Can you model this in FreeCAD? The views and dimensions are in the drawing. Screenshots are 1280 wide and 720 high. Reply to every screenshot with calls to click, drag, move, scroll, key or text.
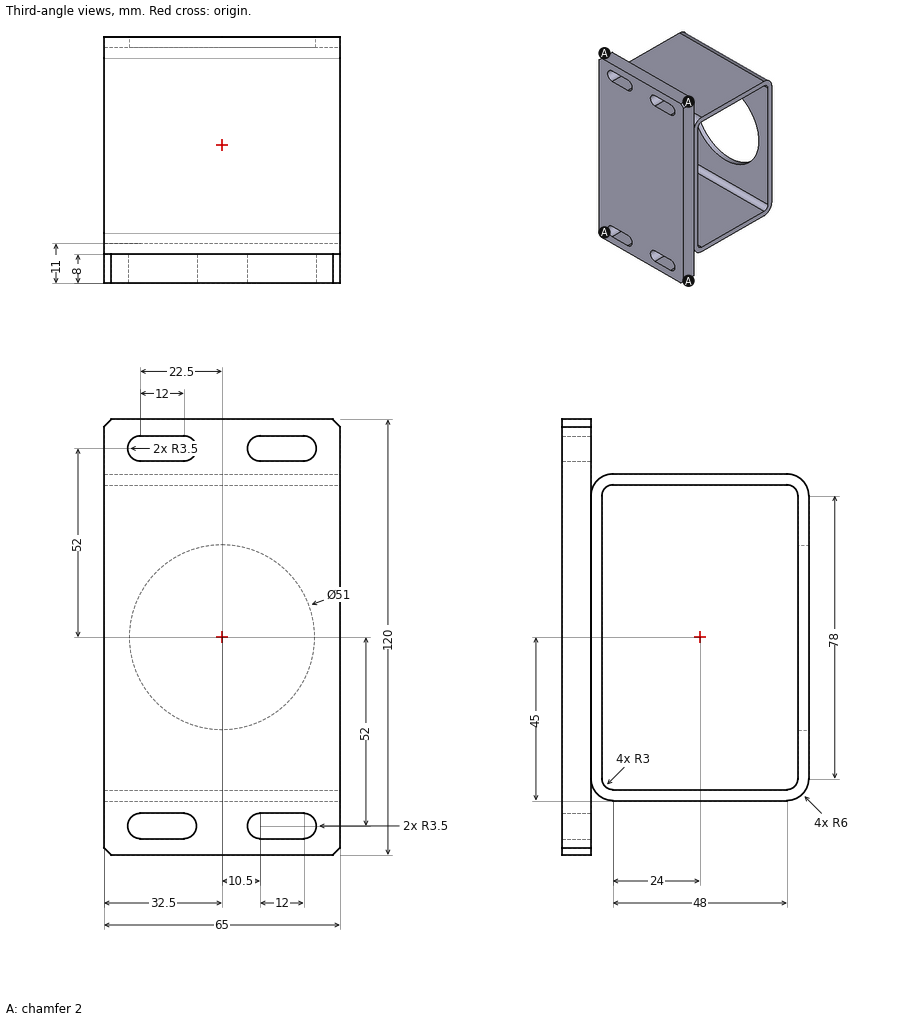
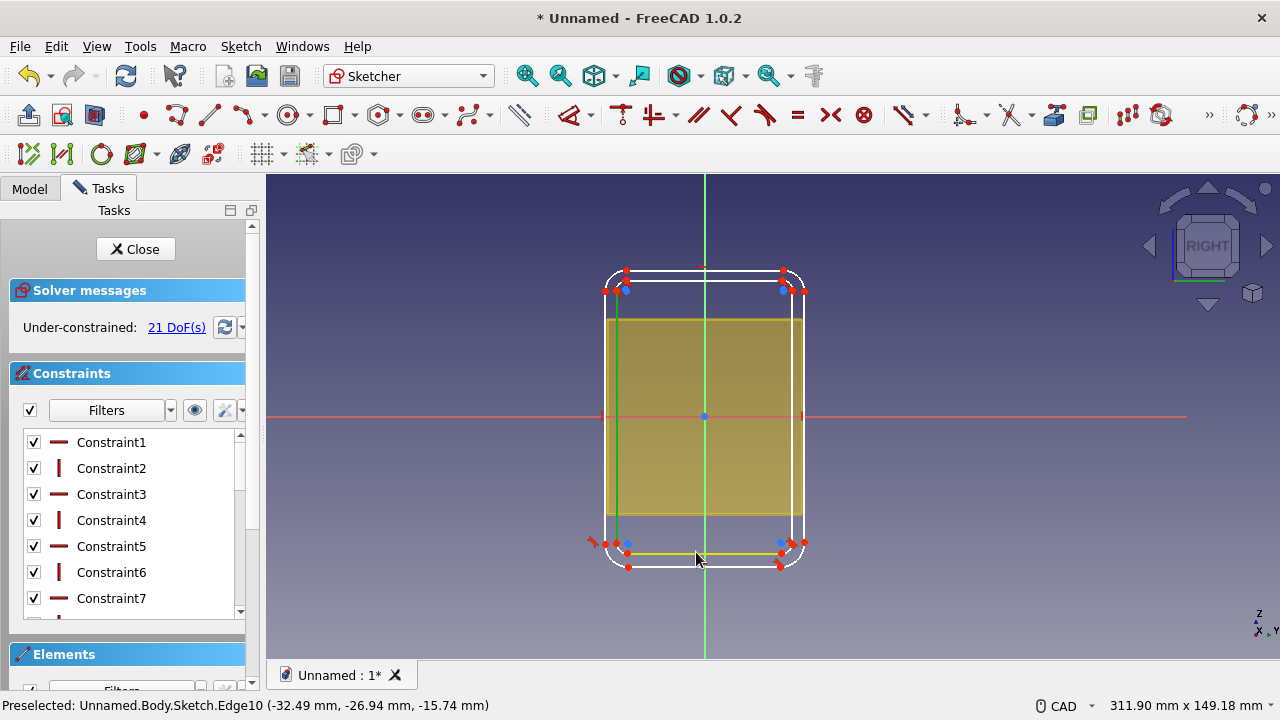
scroll(622, 282, up, 6)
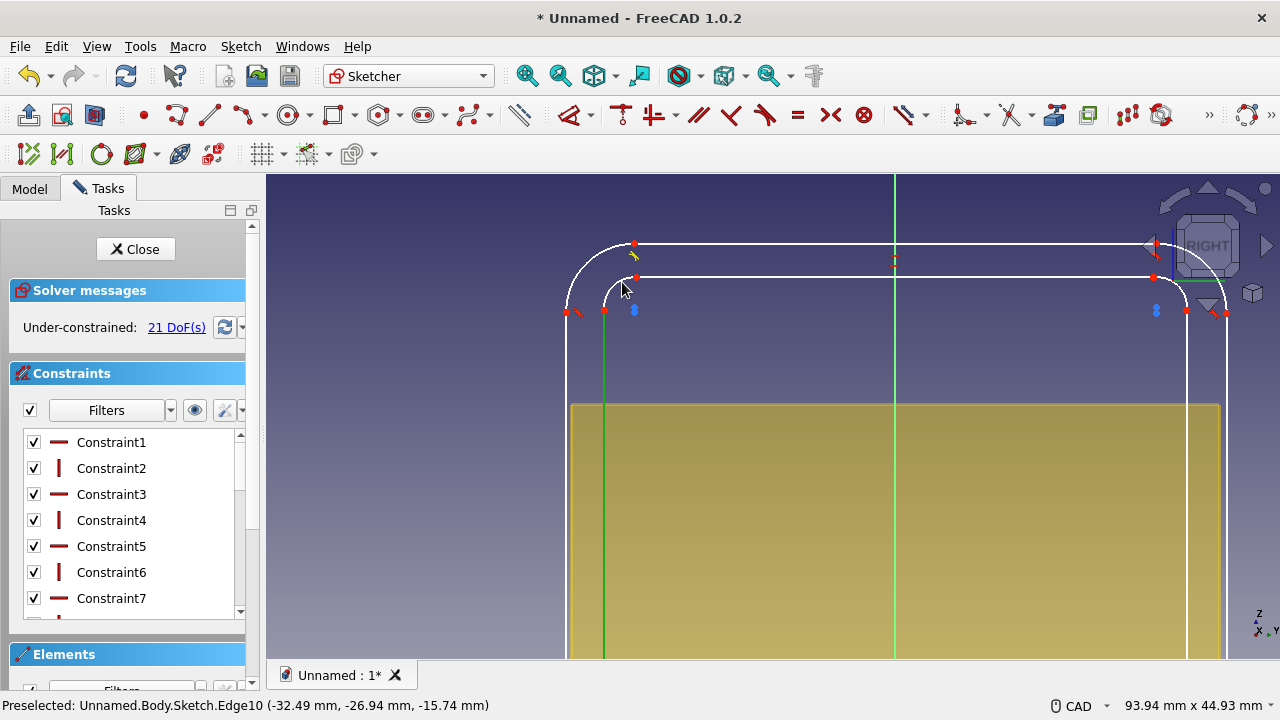
click(621, 280)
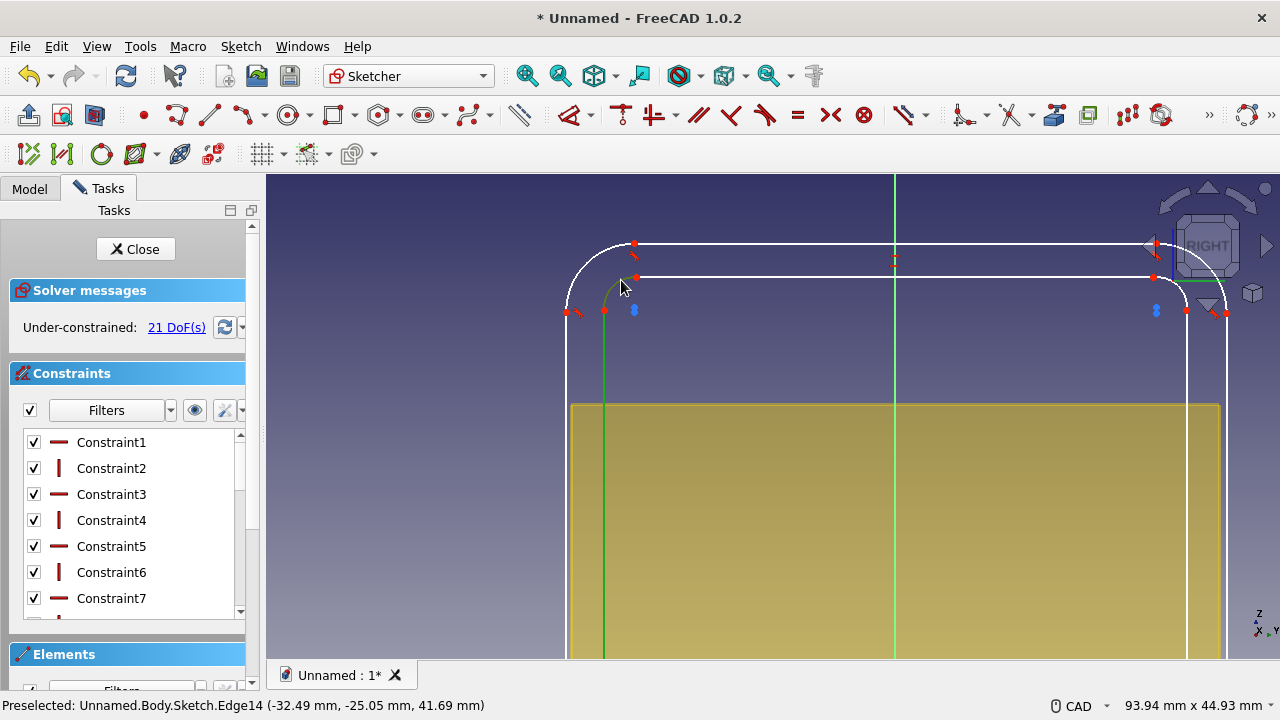
click(765, 116)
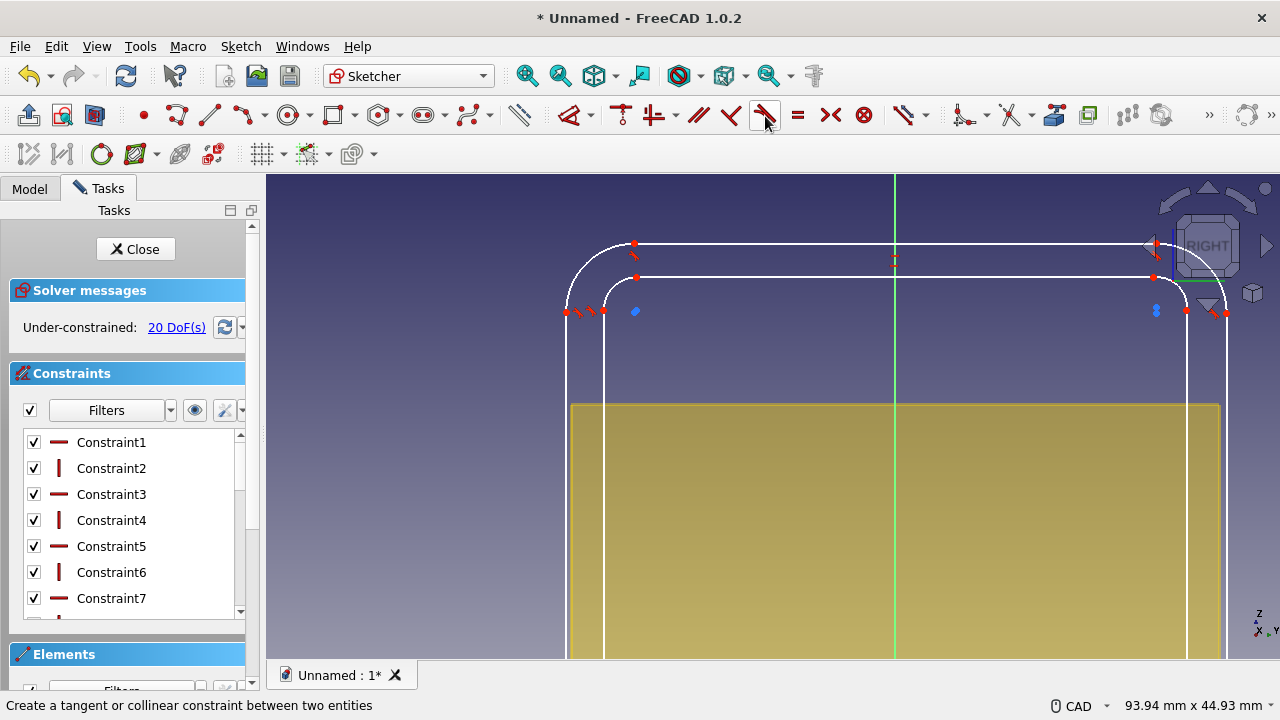
click(791, 277)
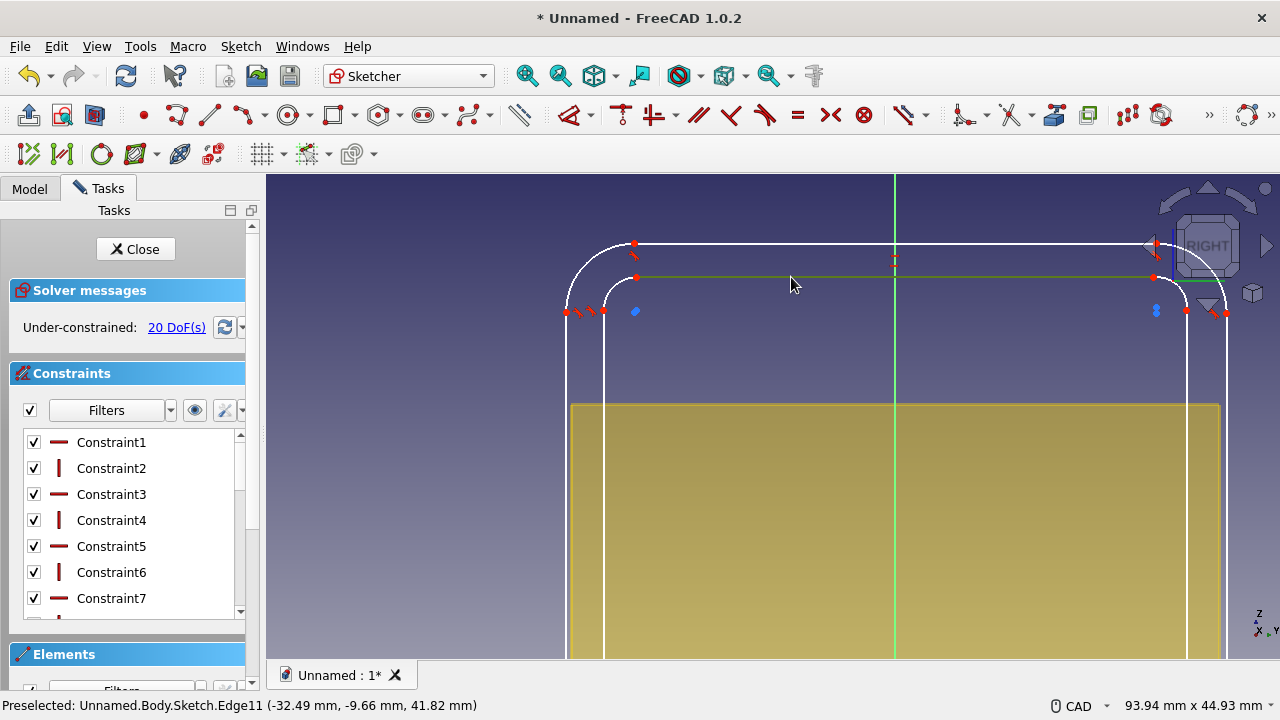
click(621, 281)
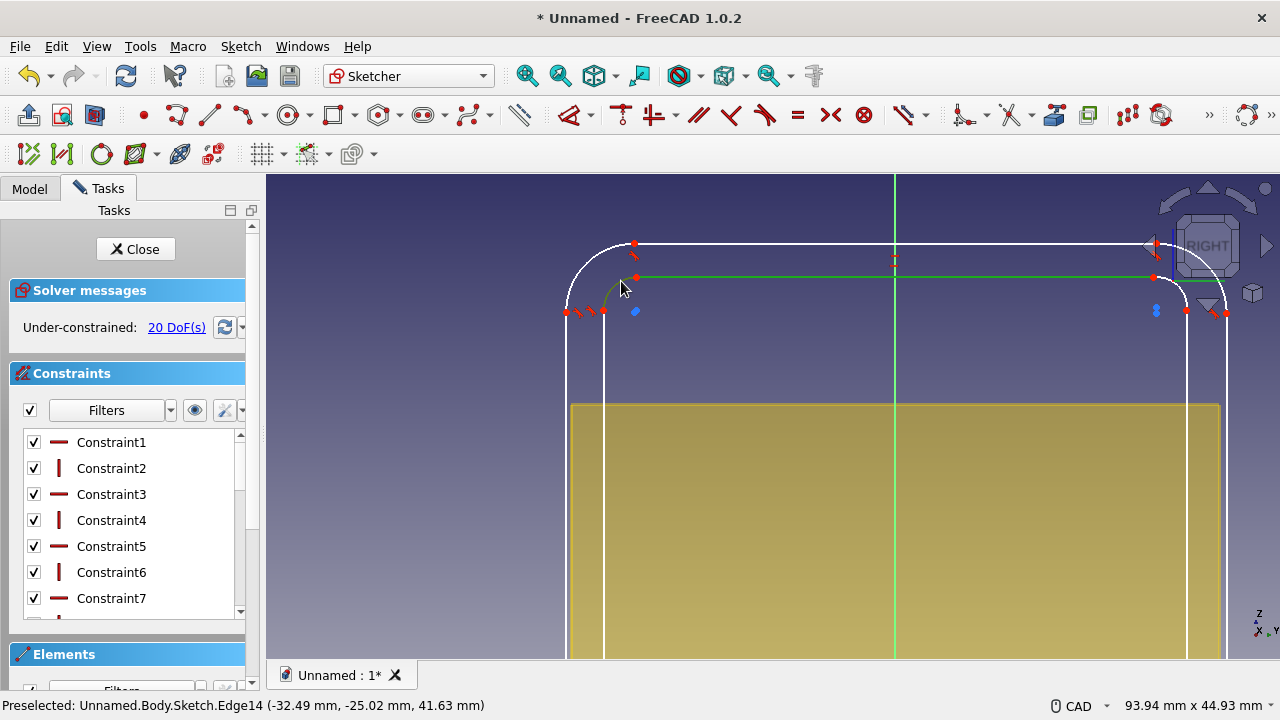
click(765, 116)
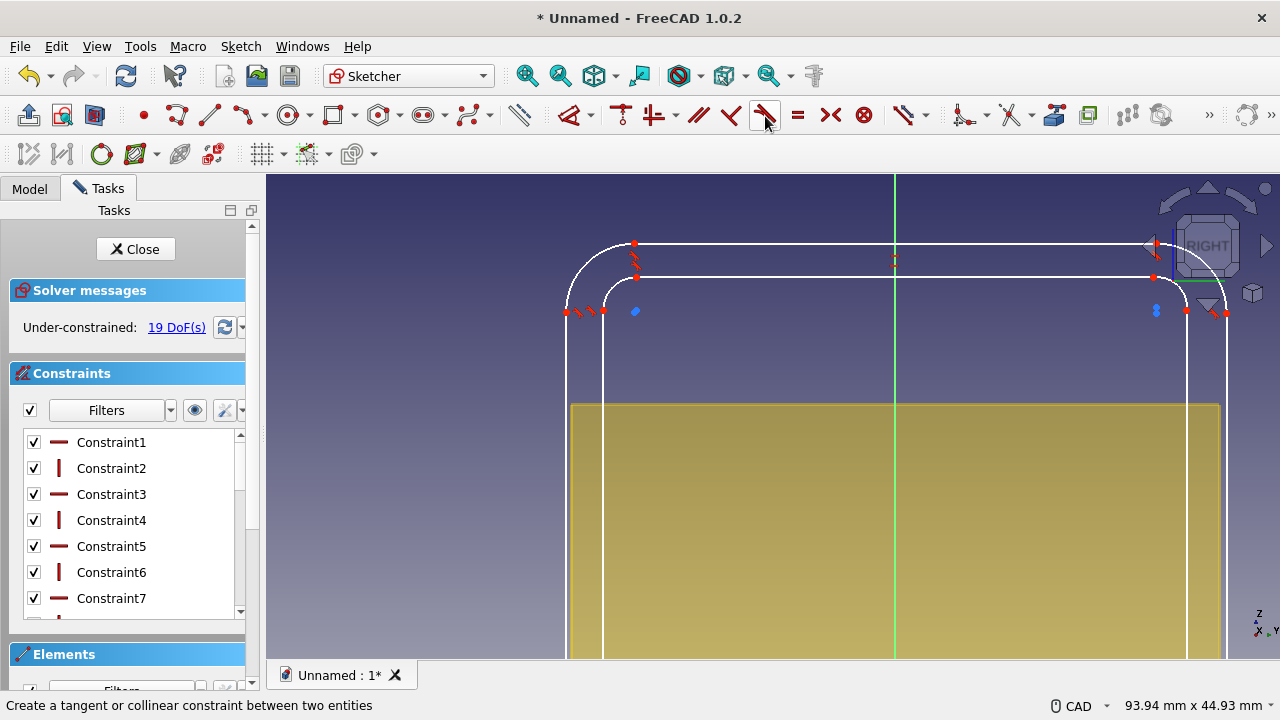
click(791, 277)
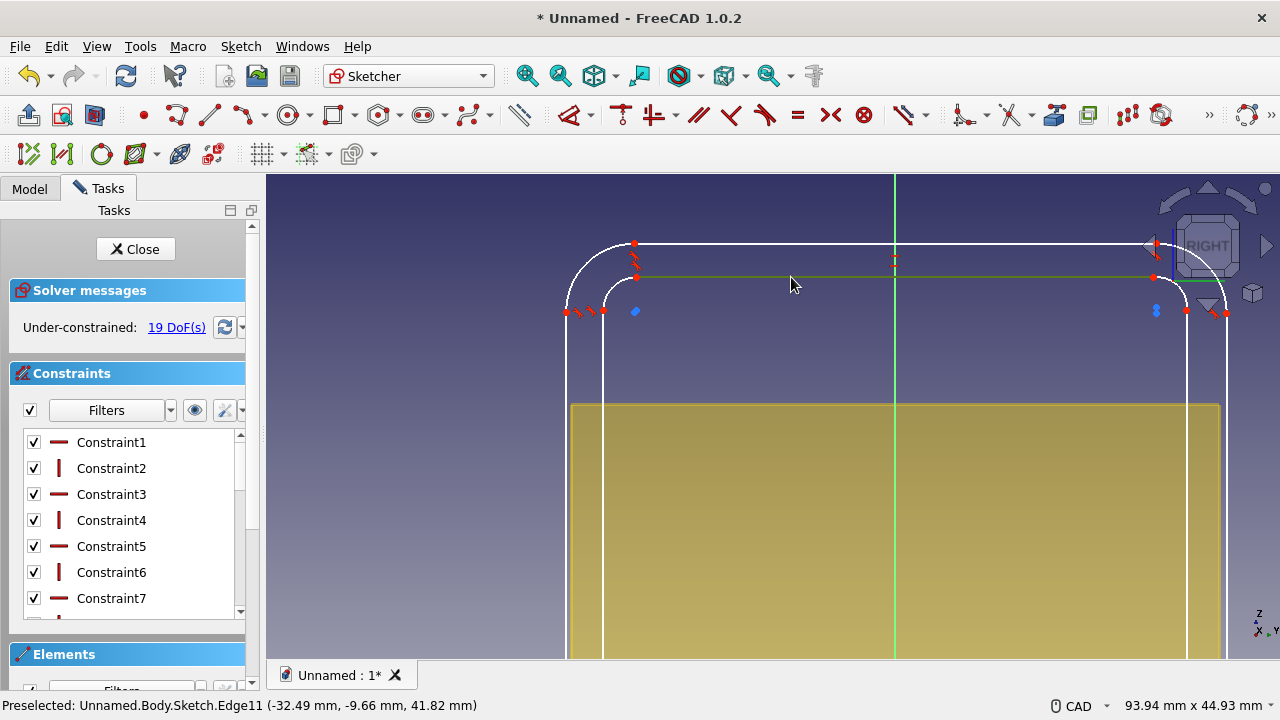
scroll(622, 282, down, 6)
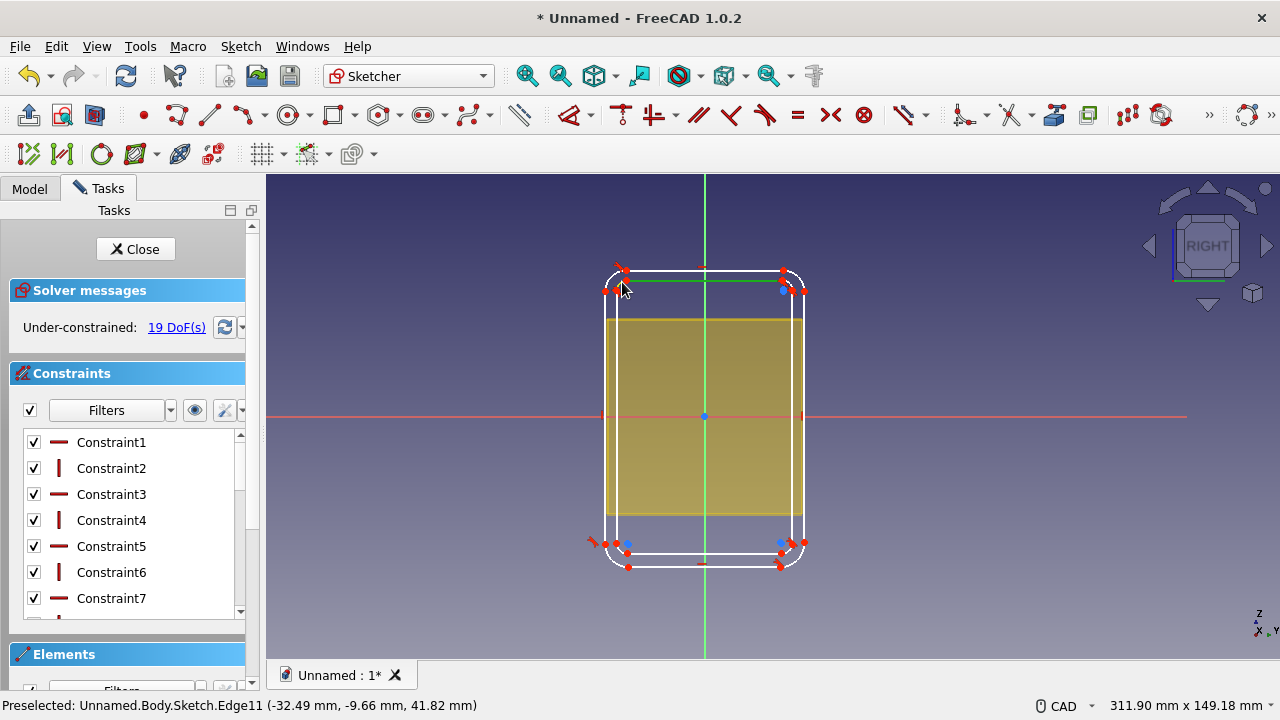
scroll(792, 286, up, 6)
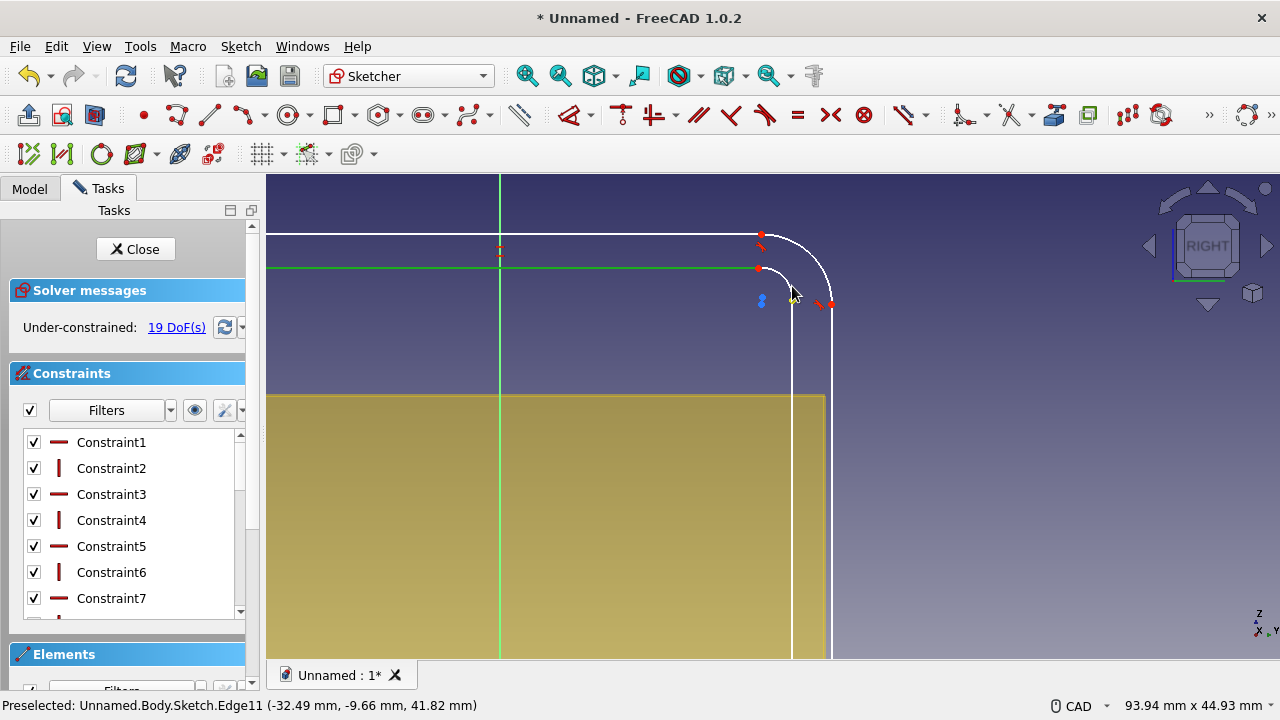
click(789, 285)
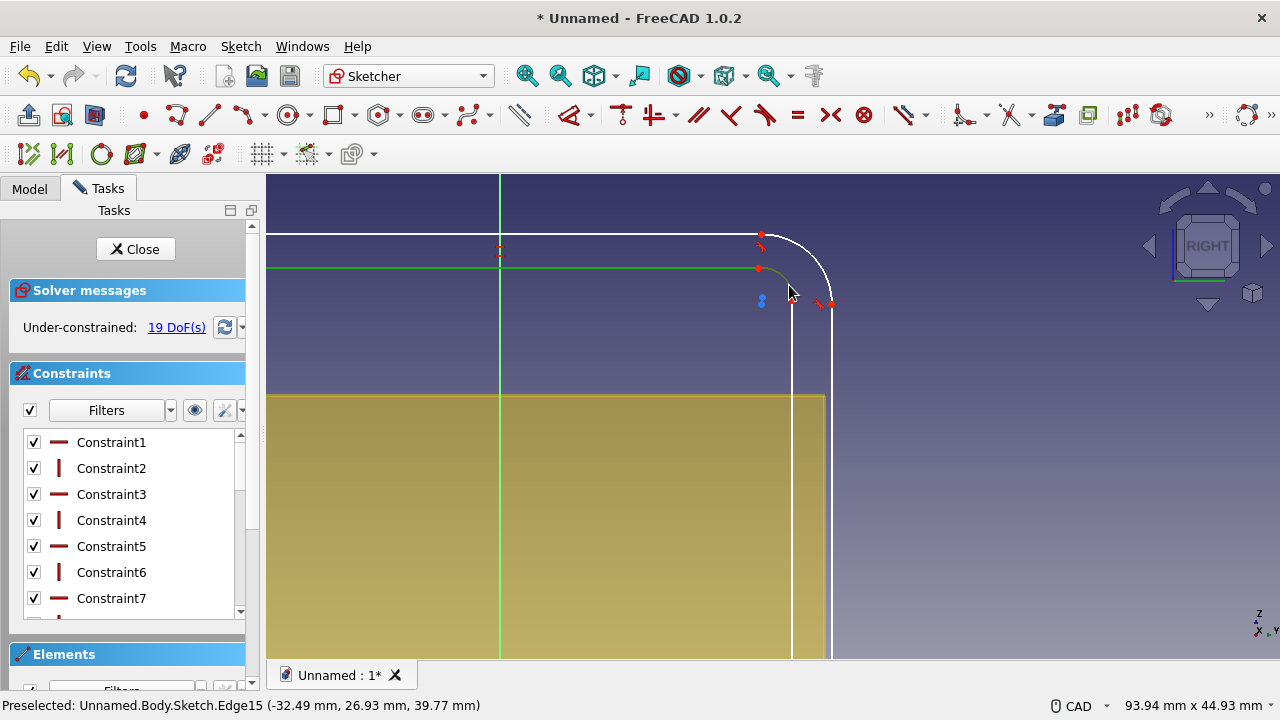
click(765, 116)